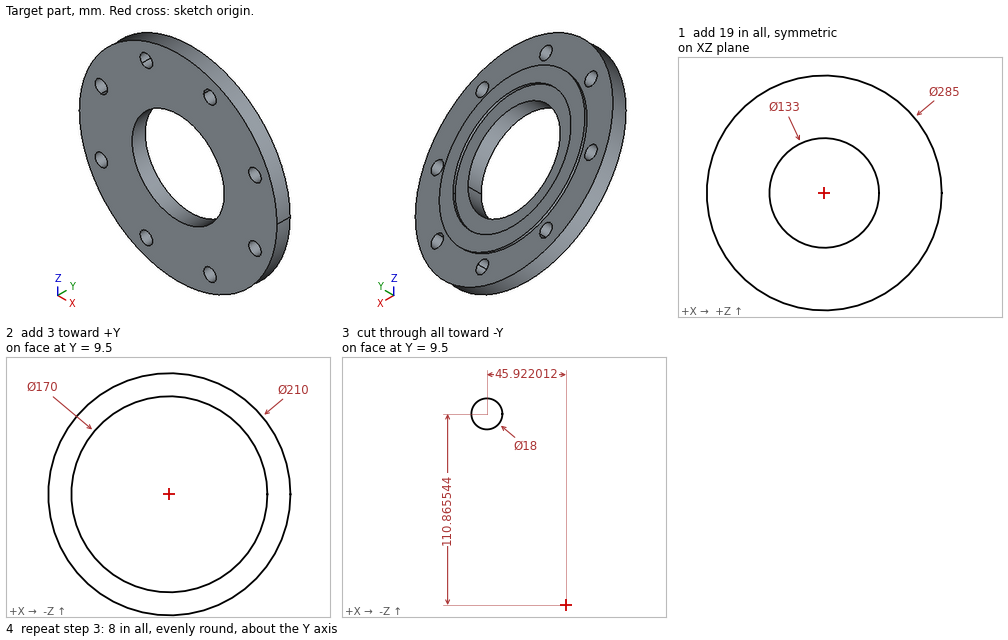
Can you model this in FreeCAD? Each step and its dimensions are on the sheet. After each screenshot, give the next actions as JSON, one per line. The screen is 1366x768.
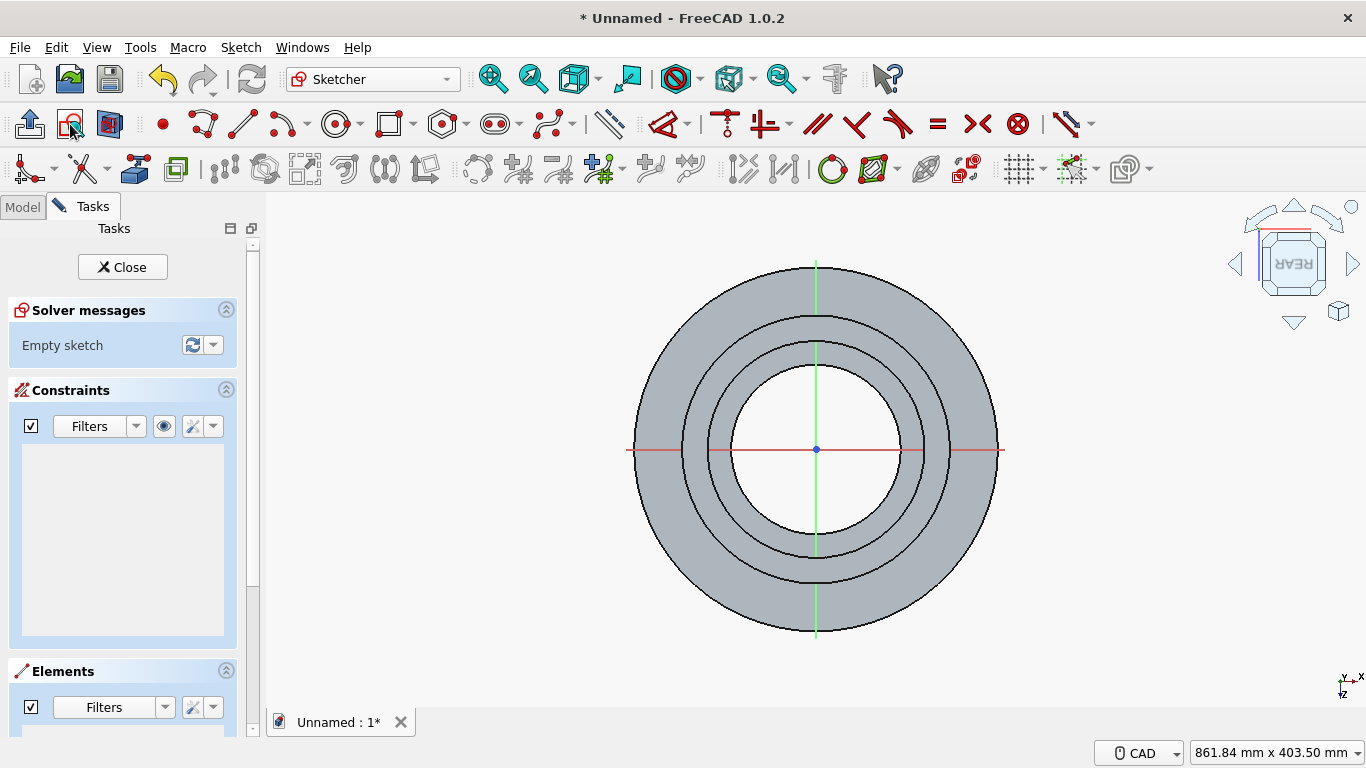
{"action": "key", "text": "q s"}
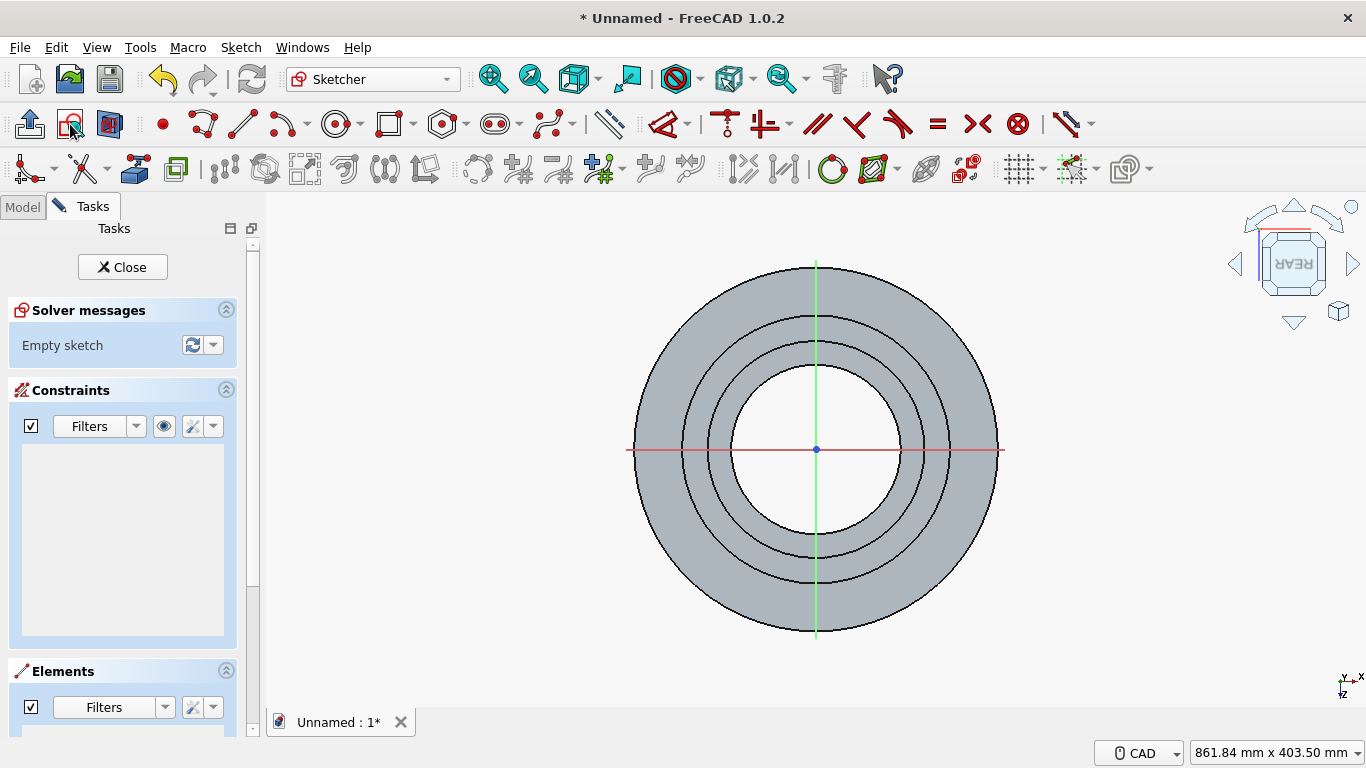
{"action": "scroll", "coordinate": [758, 297], "scroll_direction": "up", "scroll_amount": 13}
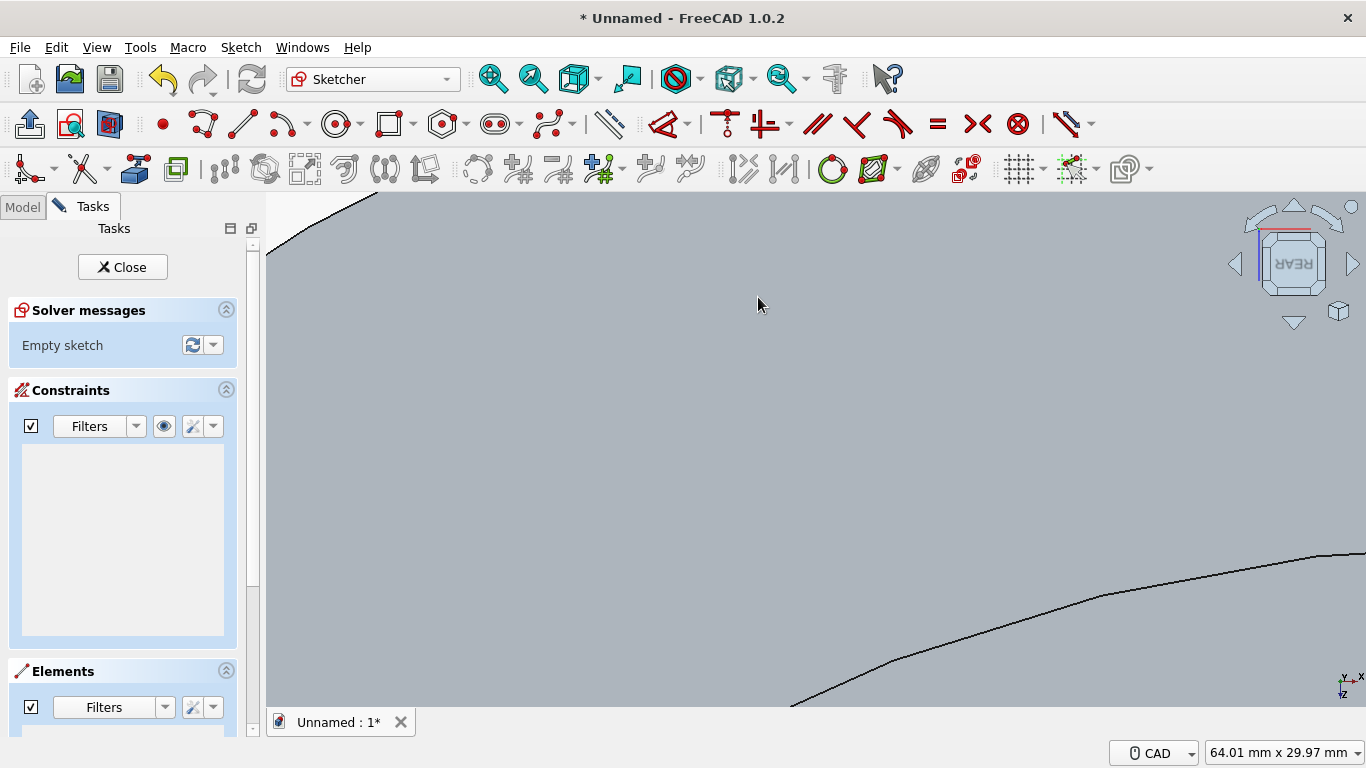
{"action": "left_click", "coordinate": [336, 124]}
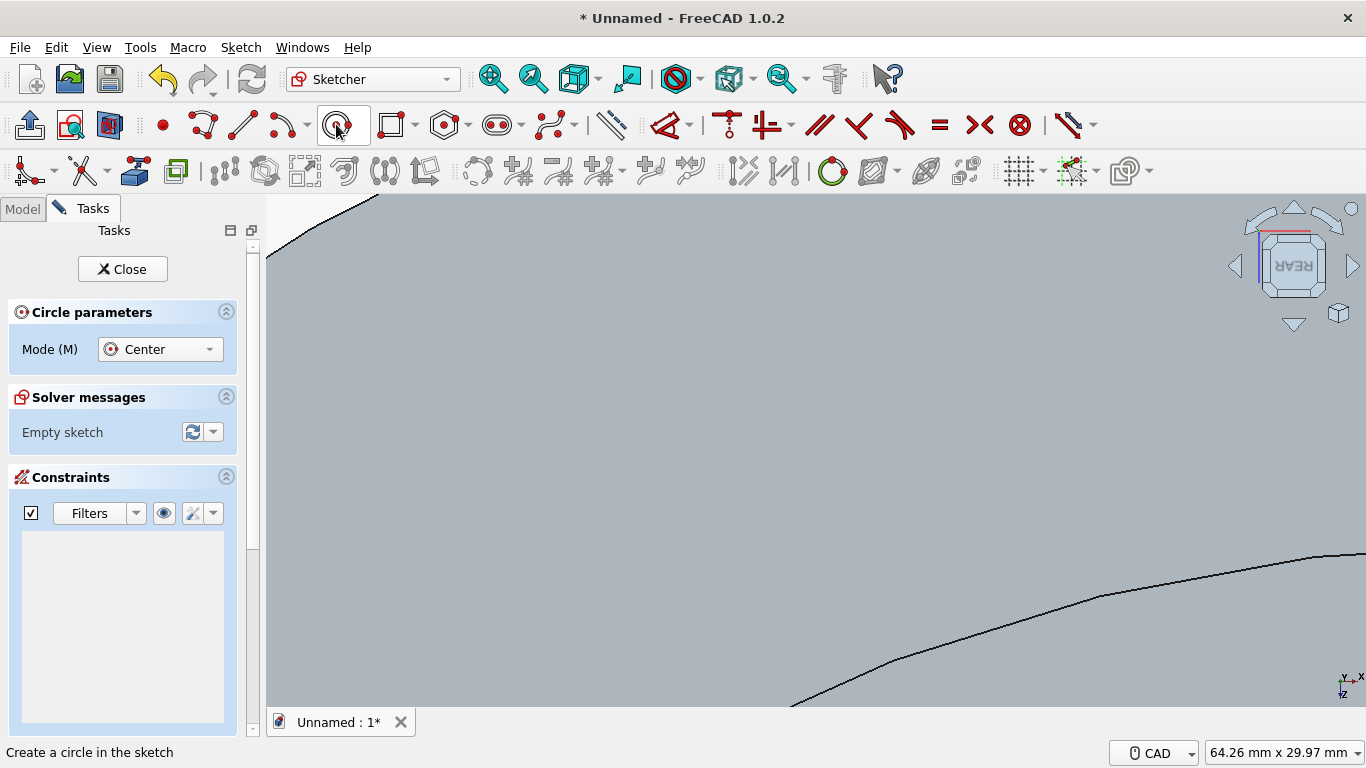
{"action": "left_click", "coordinate": [744, 444]}
{"action": "mouse_move", "coordinate": [853, 335]}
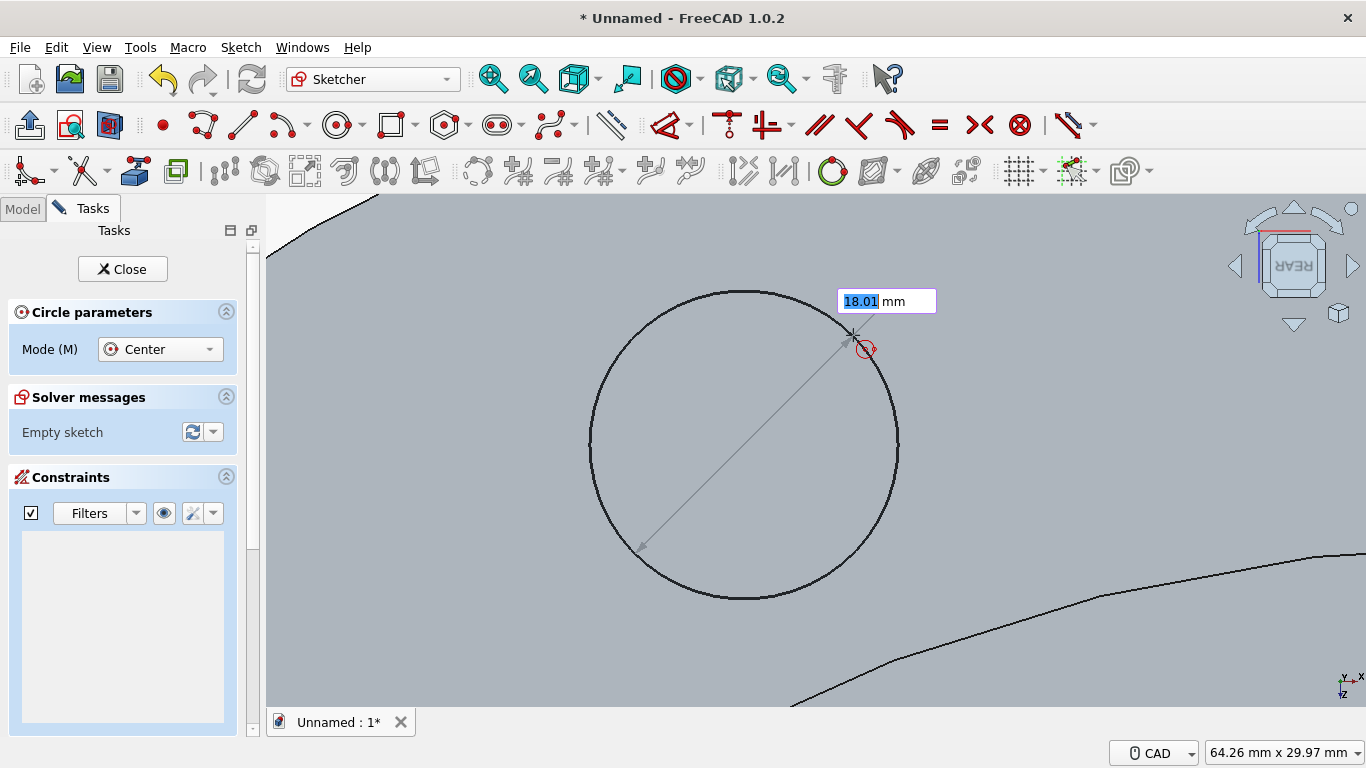
{"action": "type", "text": "18"}
{"action": "key", "text": "Return"}
{"action": "key", "text": "Escape"}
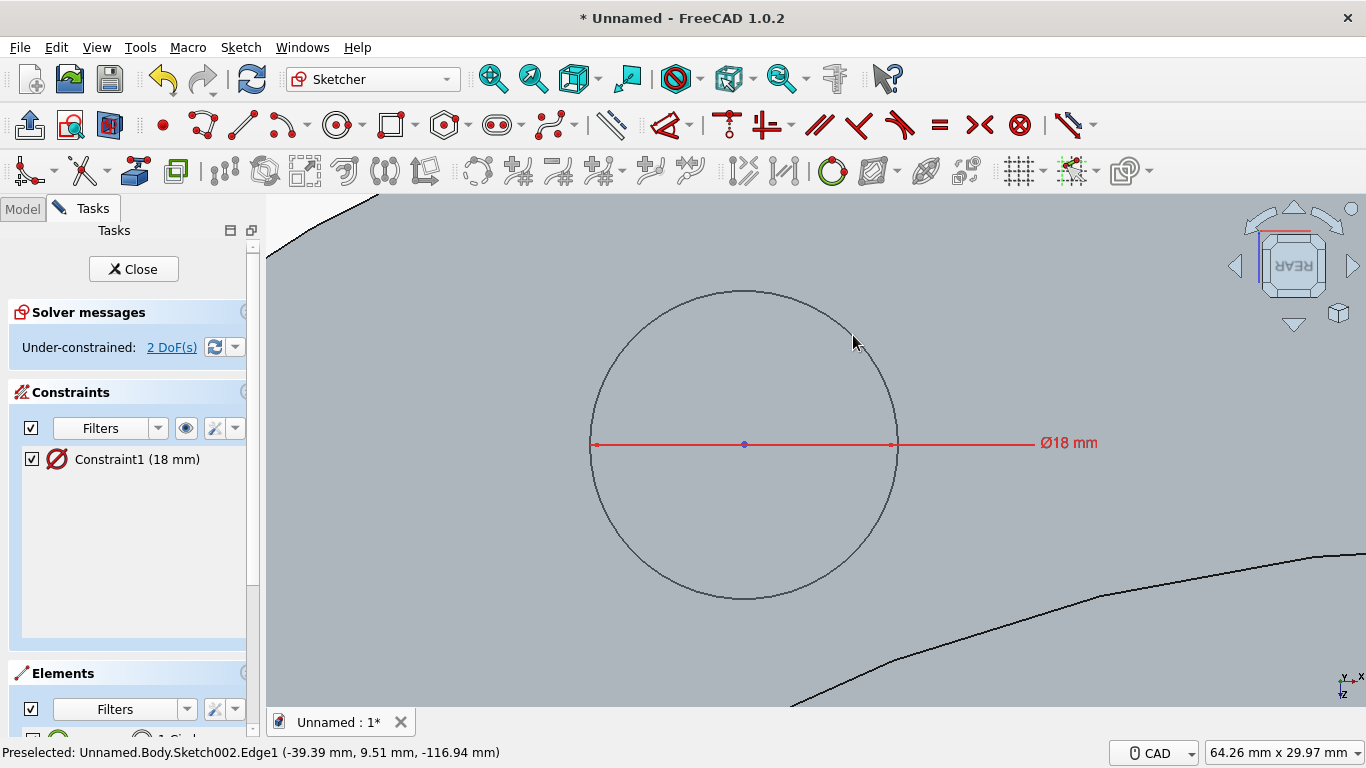
{"action": "left_click", "coordinate": [744, 445]}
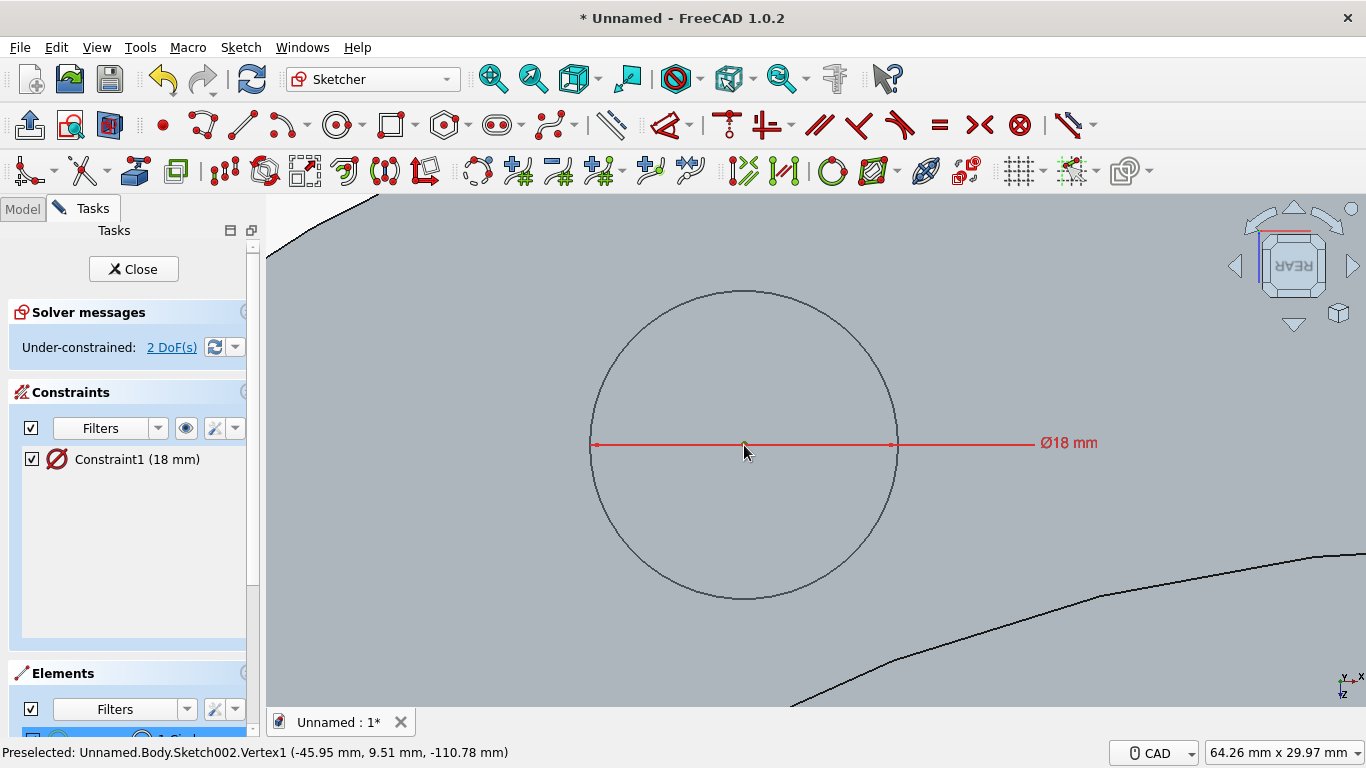
{"action": "left_click", "coordinate": [692, 126]}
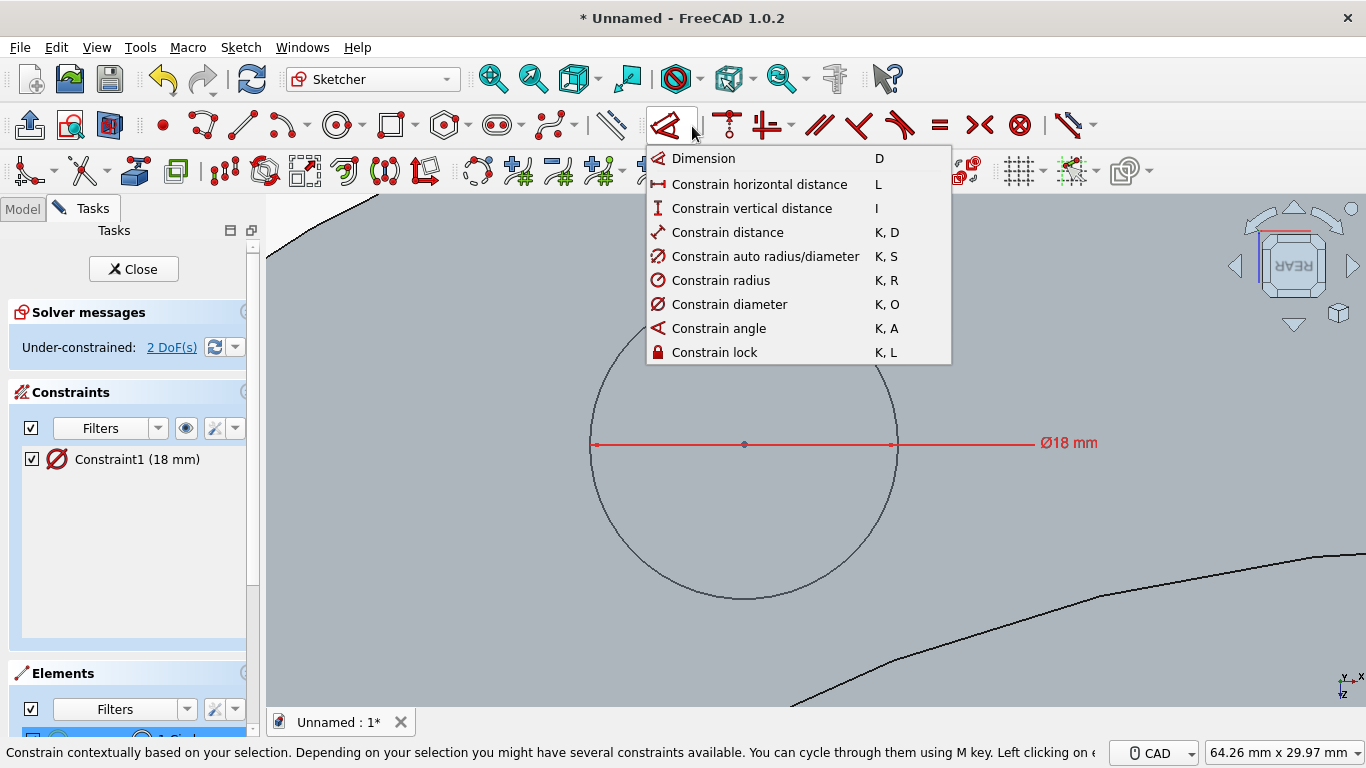
{"action": "left_click", "coordinate": [799, 184]}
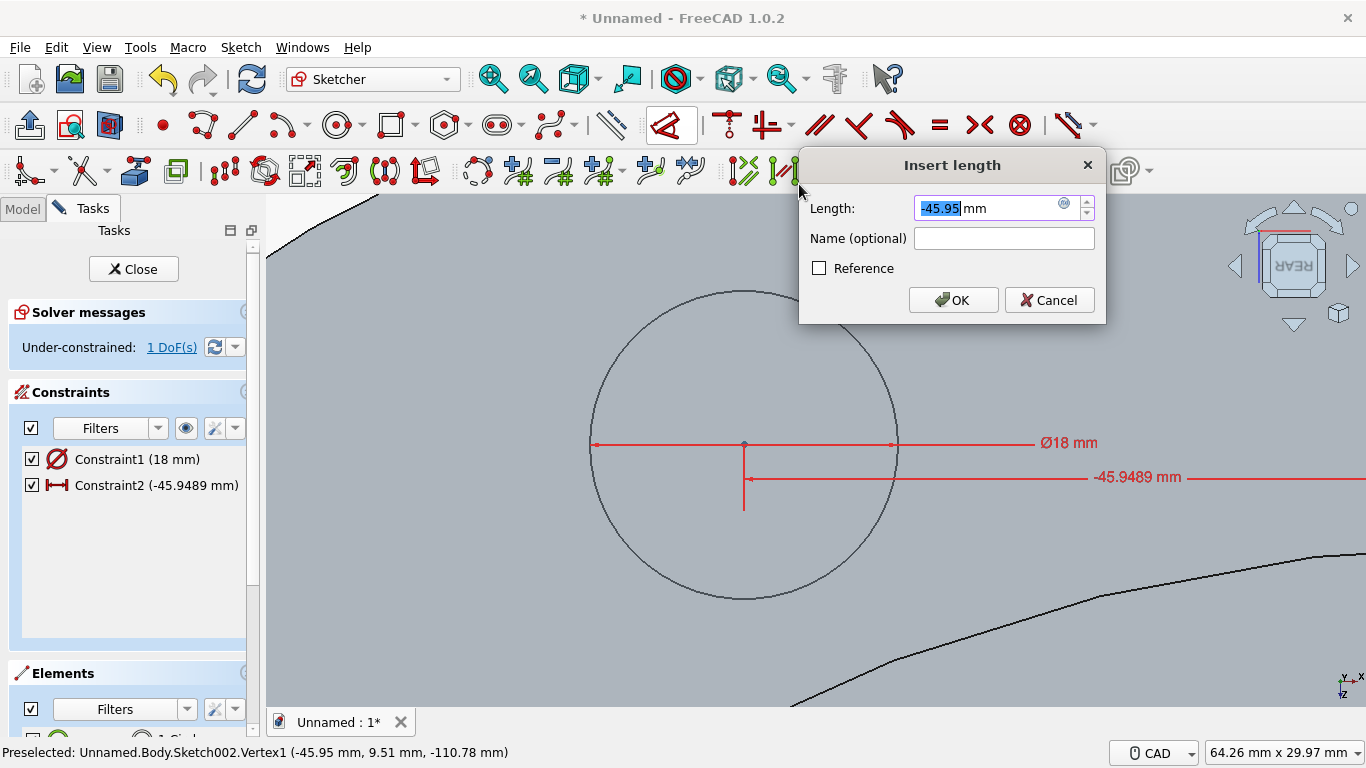
{"action": "type", "text": "-45.922012"}
{"action": "key", "text": "Return"}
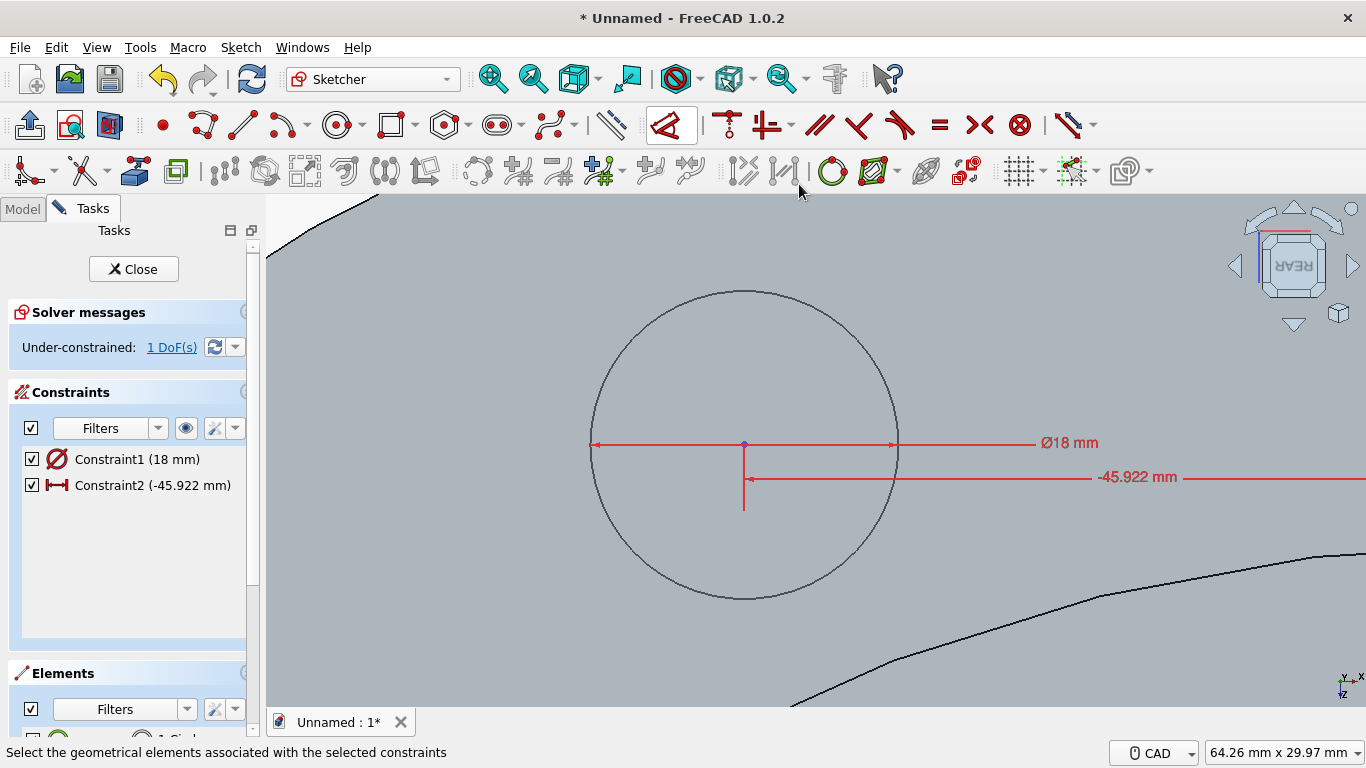
{"action": "left_click", "coordinate": [744, 445]}